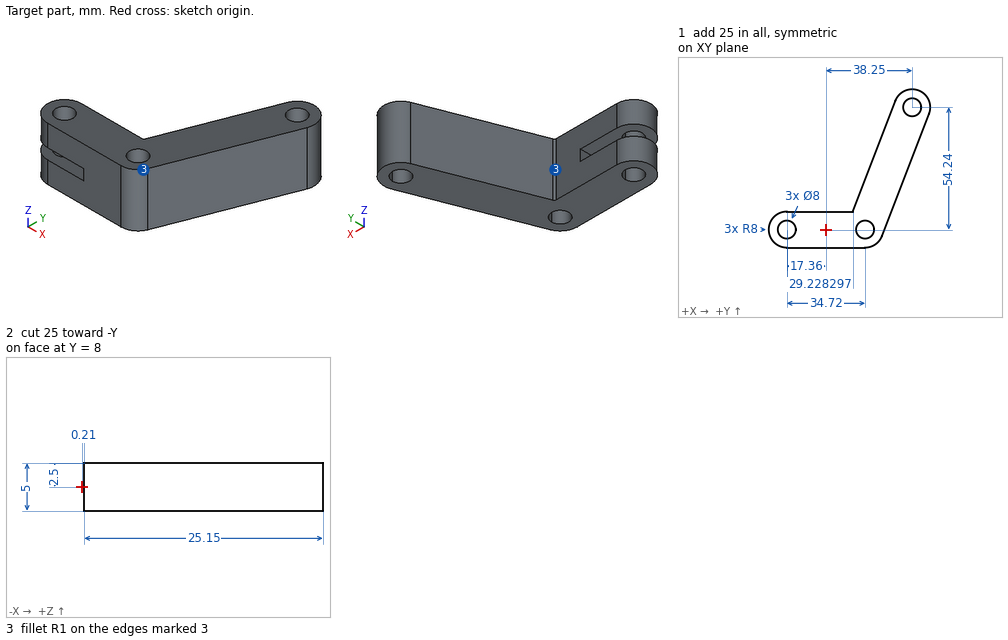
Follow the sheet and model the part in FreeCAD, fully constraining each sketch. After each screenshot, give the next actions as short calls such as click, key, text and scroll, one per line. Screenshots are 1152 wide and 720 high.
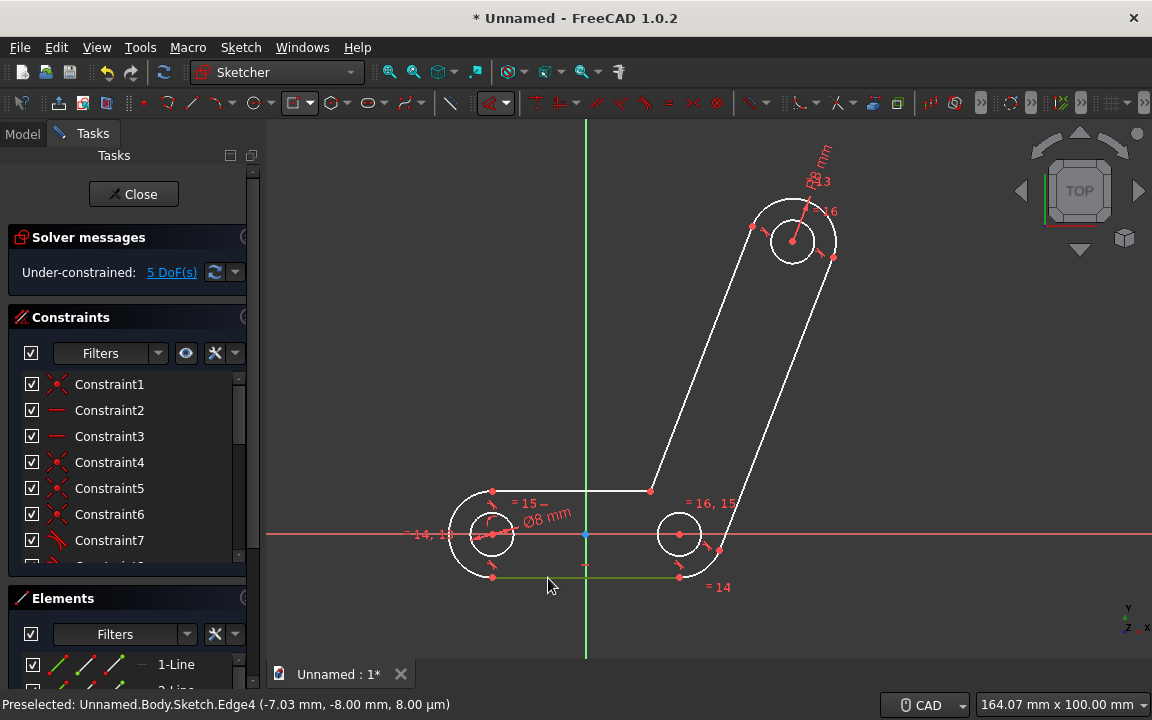
key(l)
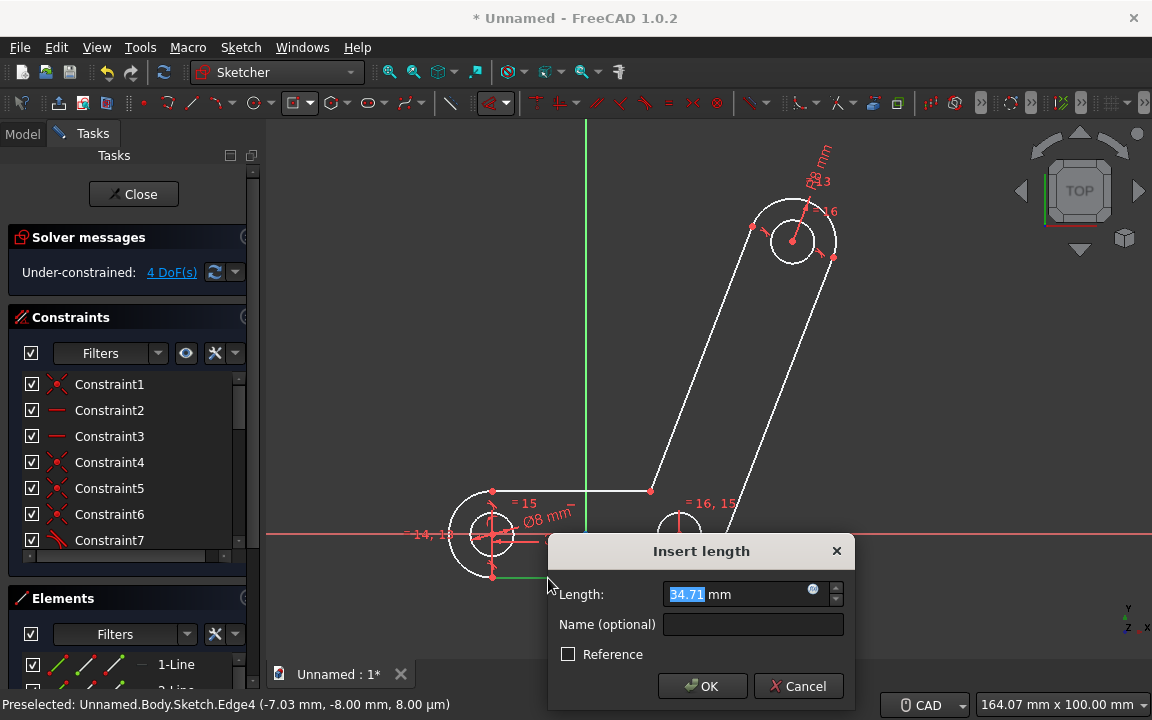
text(34.72)
key(Return)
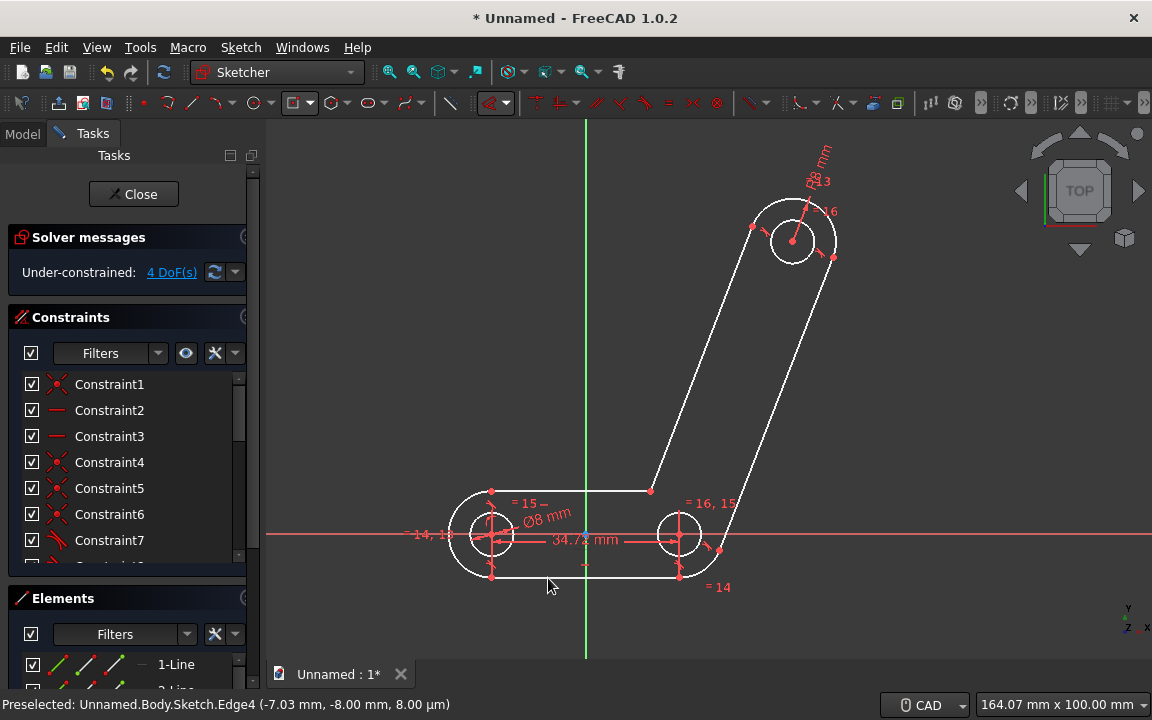
click(492, 534)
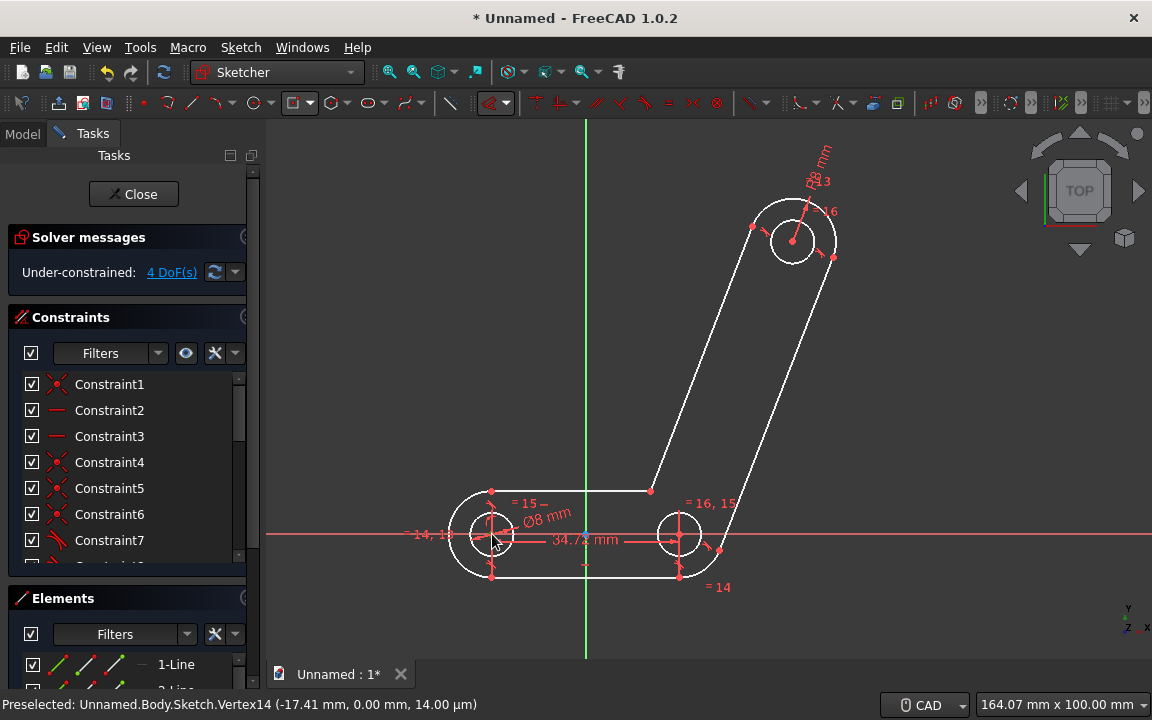
click(508, 104)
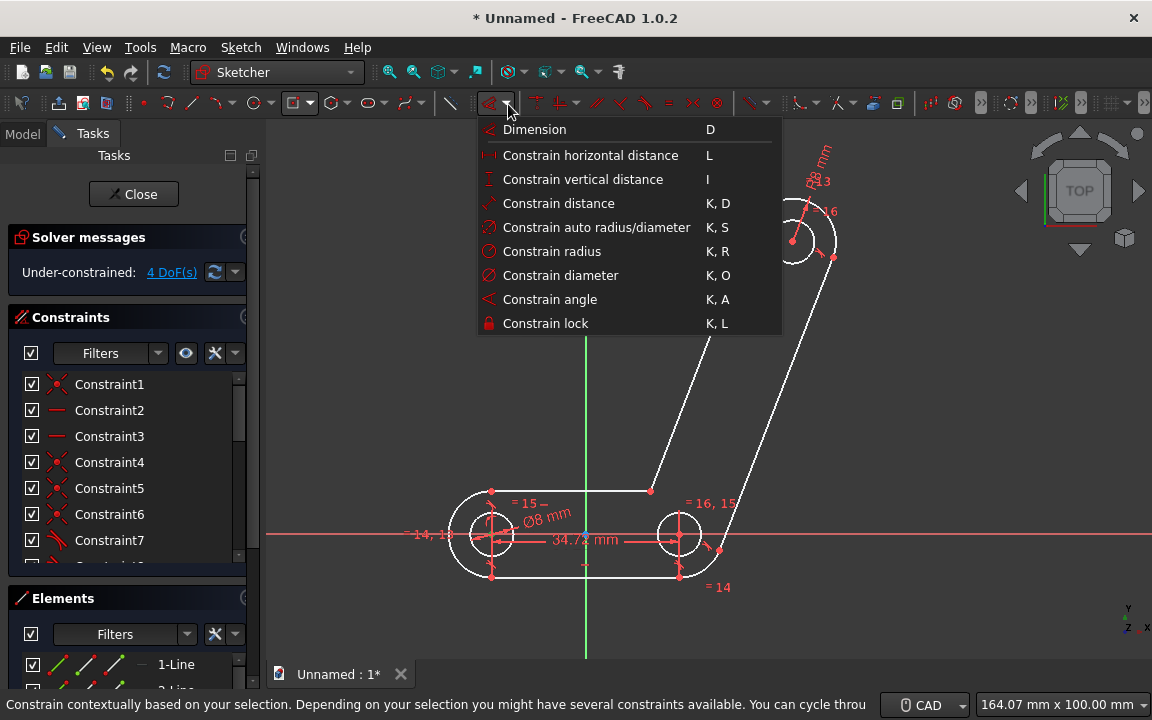
click(630, 155)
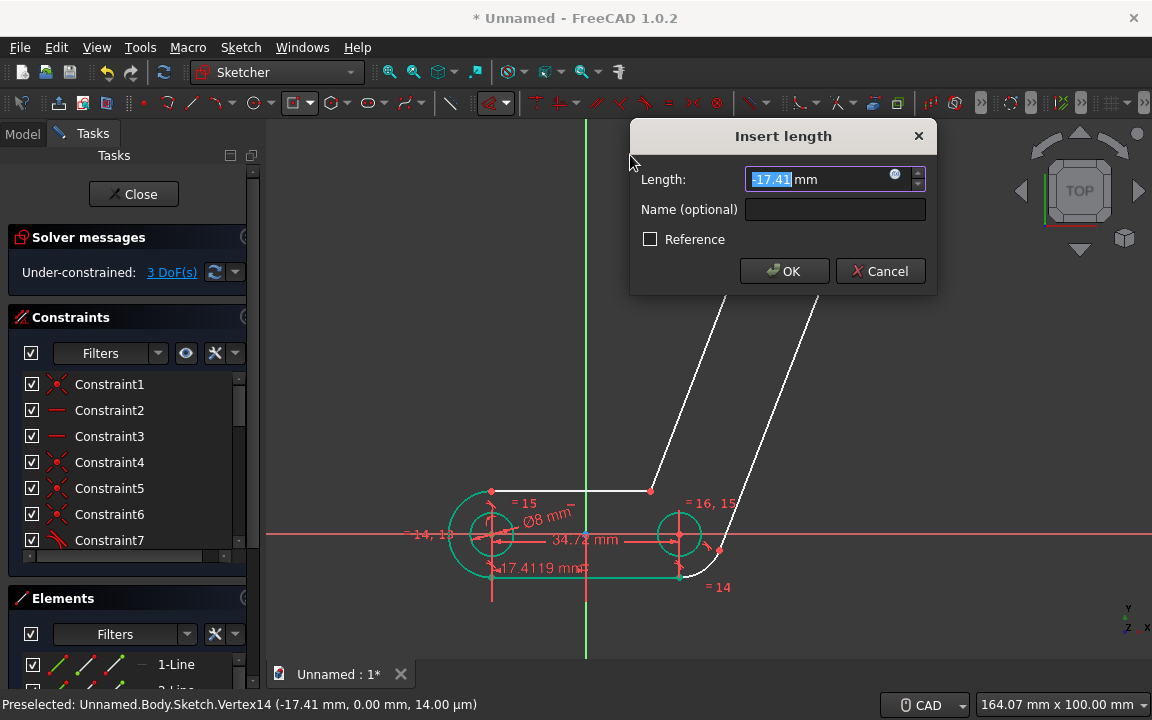
text(-17.36)
key(Return)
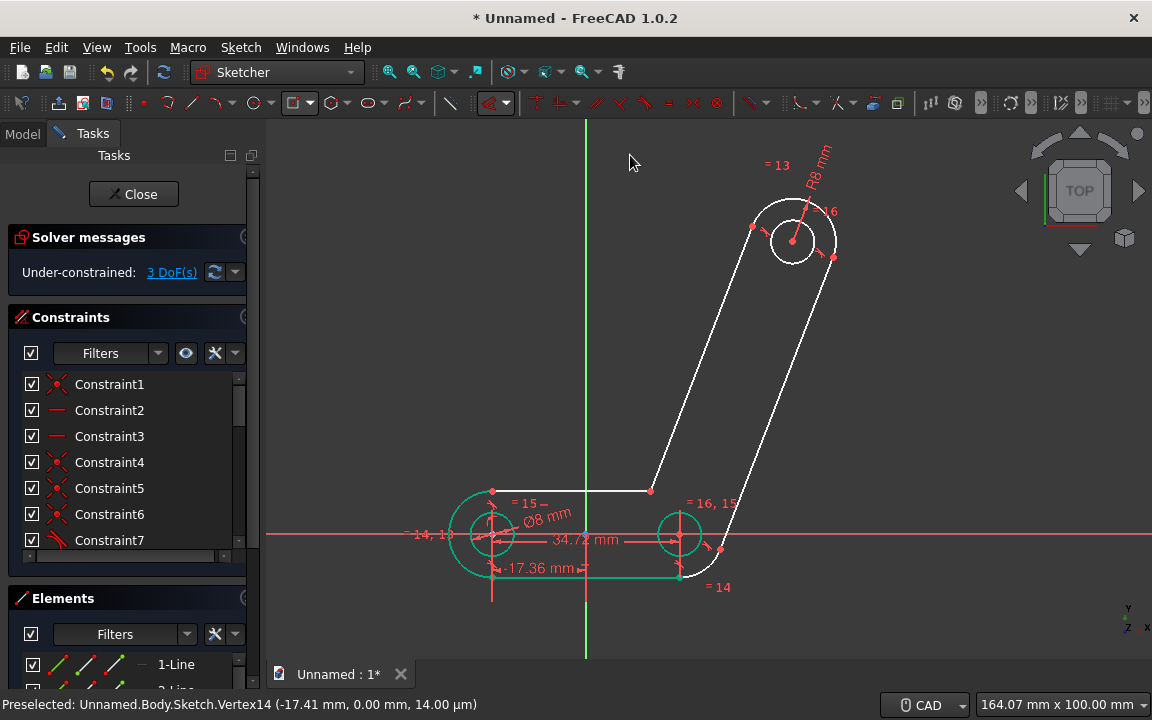
click(793, 242)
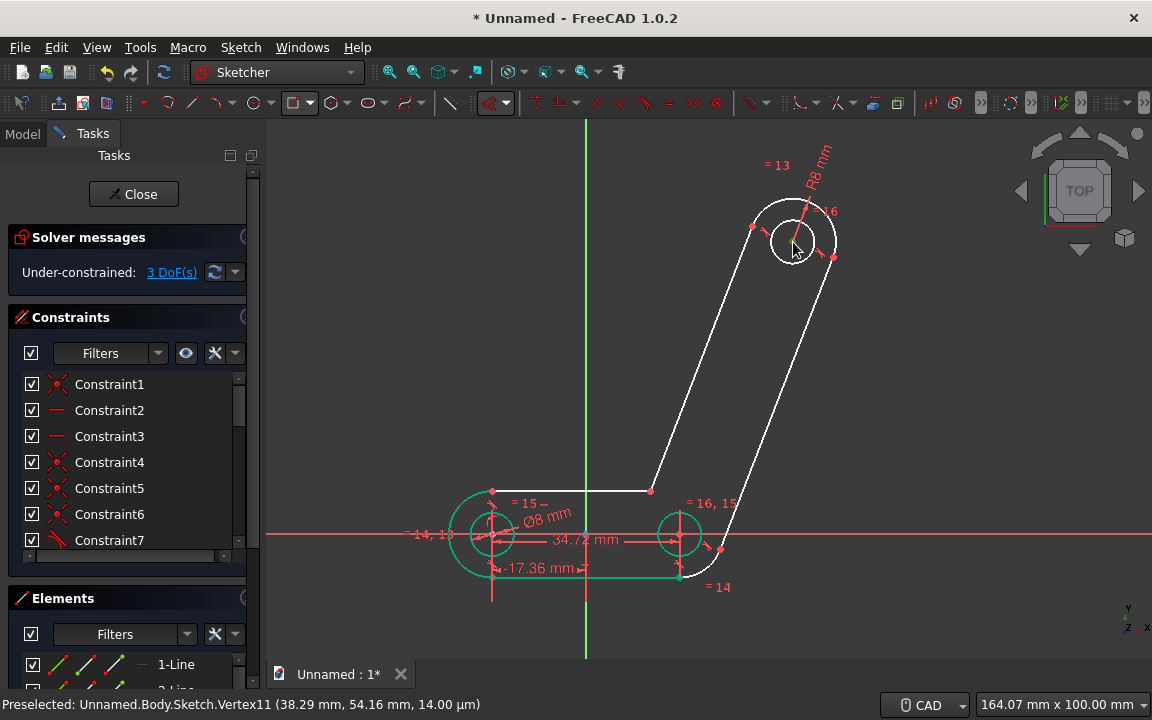
key(l)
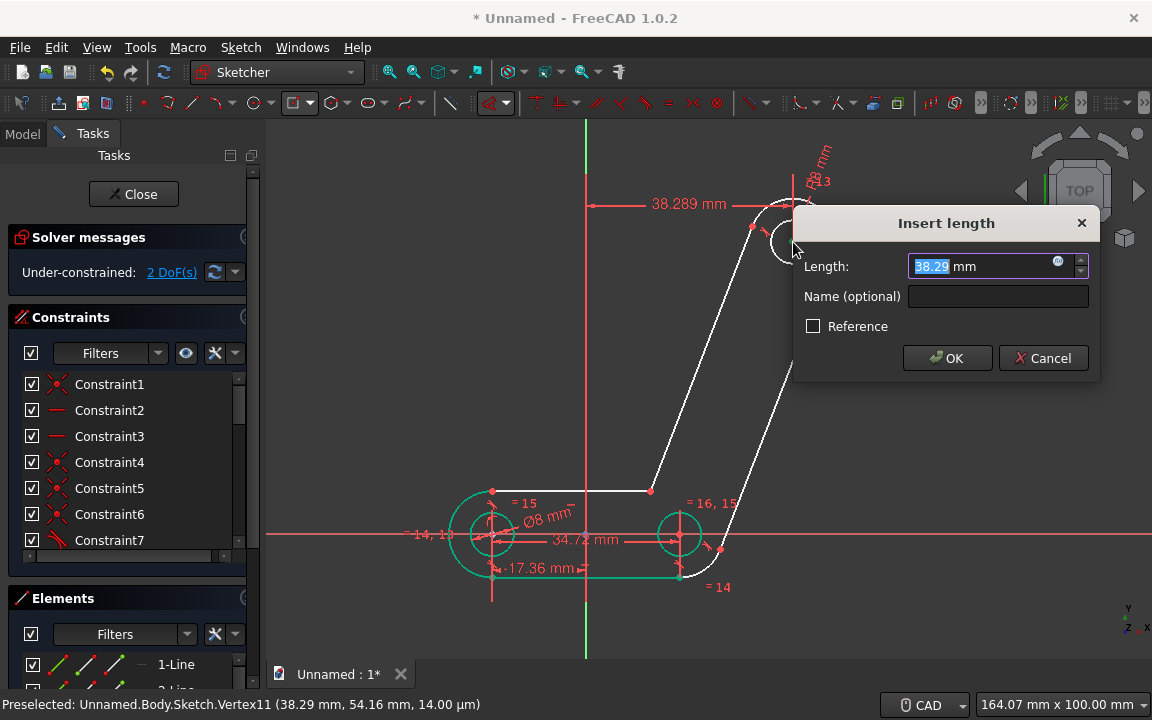
text(38.25)
key(Return)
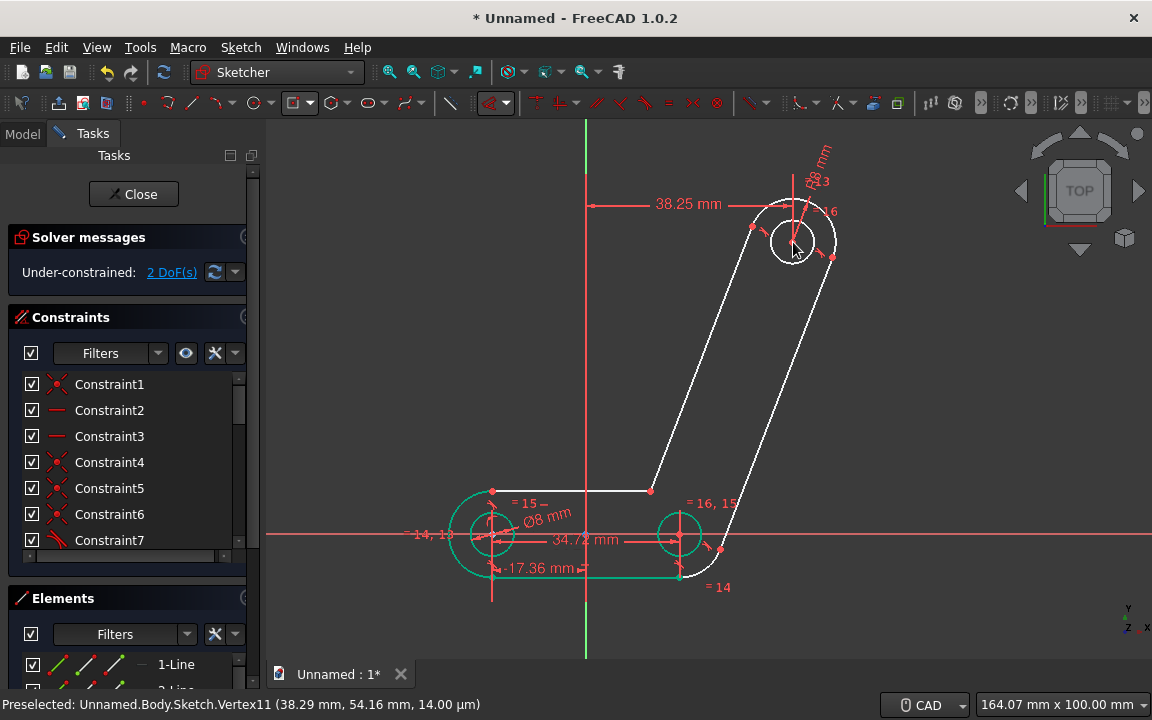
click(793, 242)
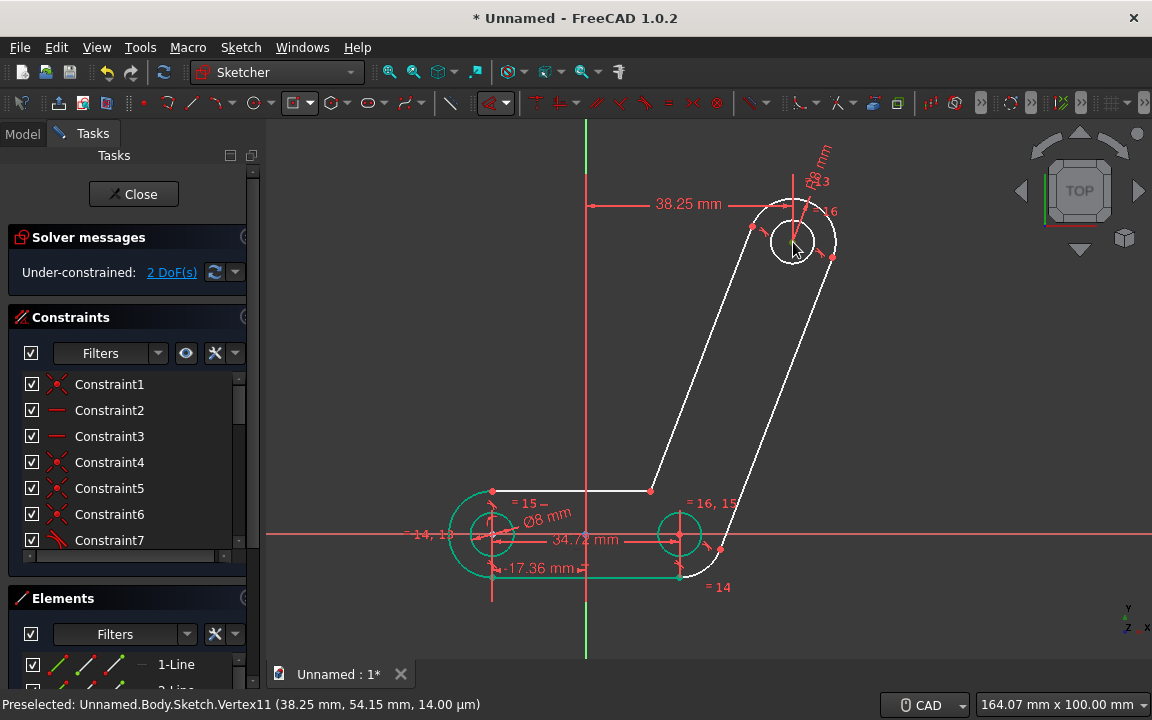
key(i)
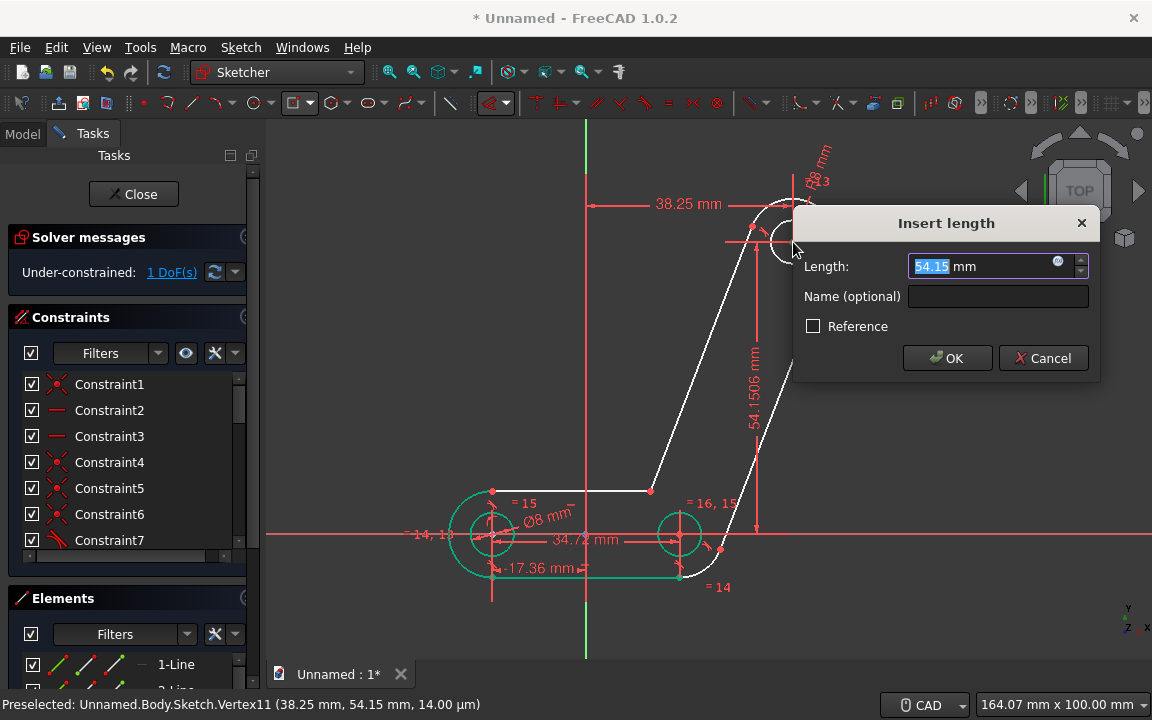
text(54.24)
key(Return)